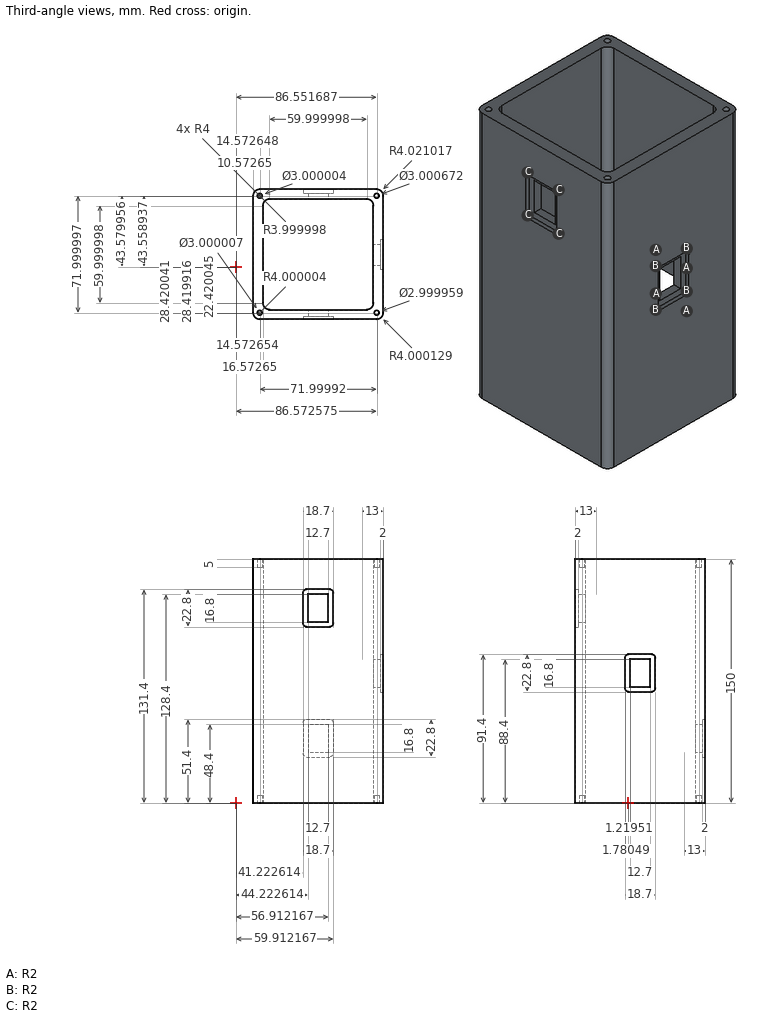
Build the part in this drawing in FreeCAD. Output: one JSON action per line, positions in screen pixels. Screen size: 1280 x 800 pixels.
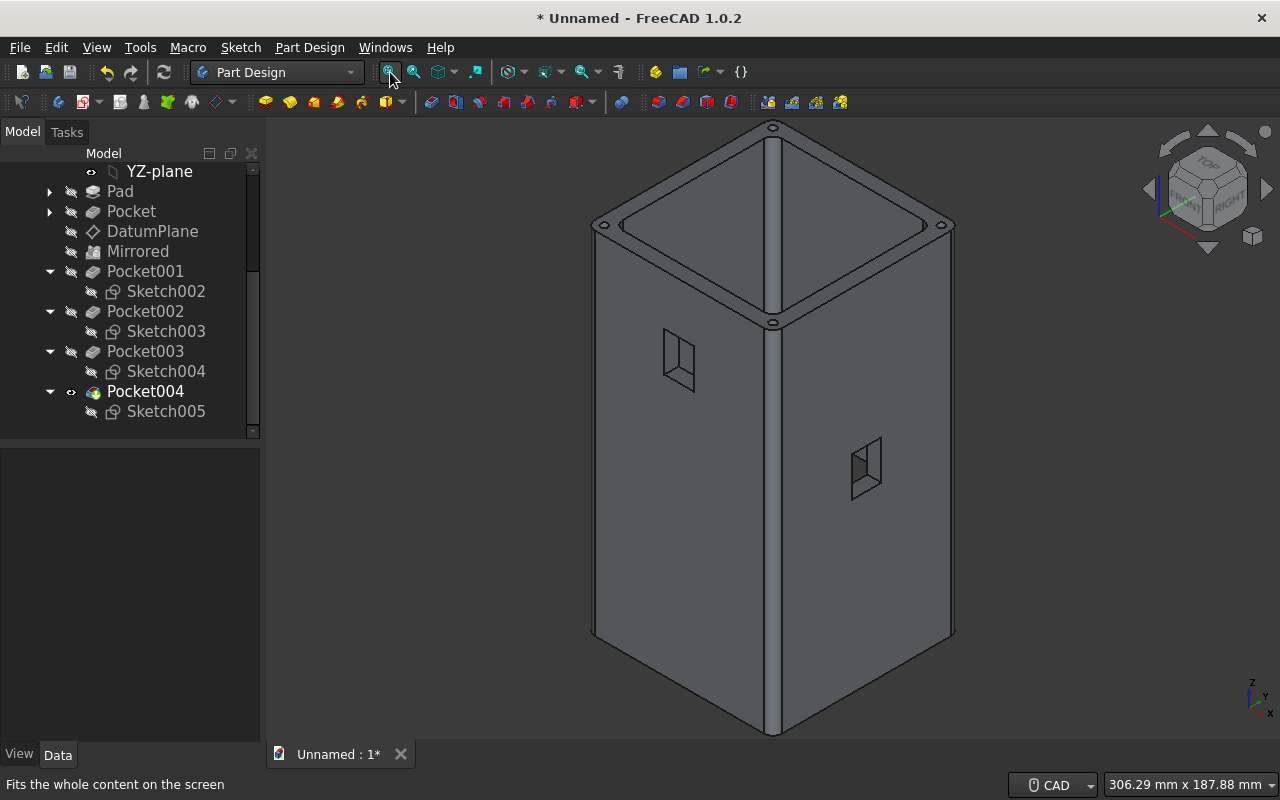
{"action": "key", "text": "v f"}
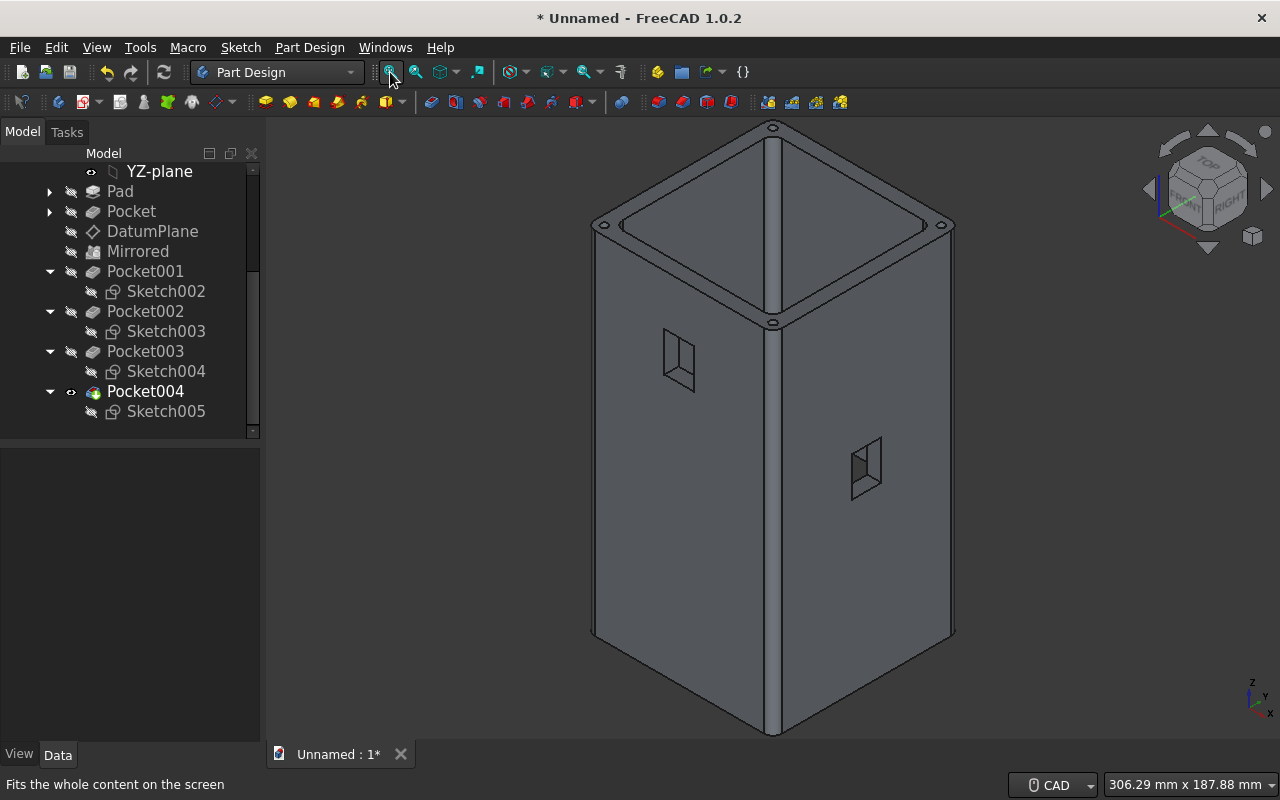
{"action": "scroll", "coordinate": [886, 512], "scroll_direction": "up", "scroll_amount": 9}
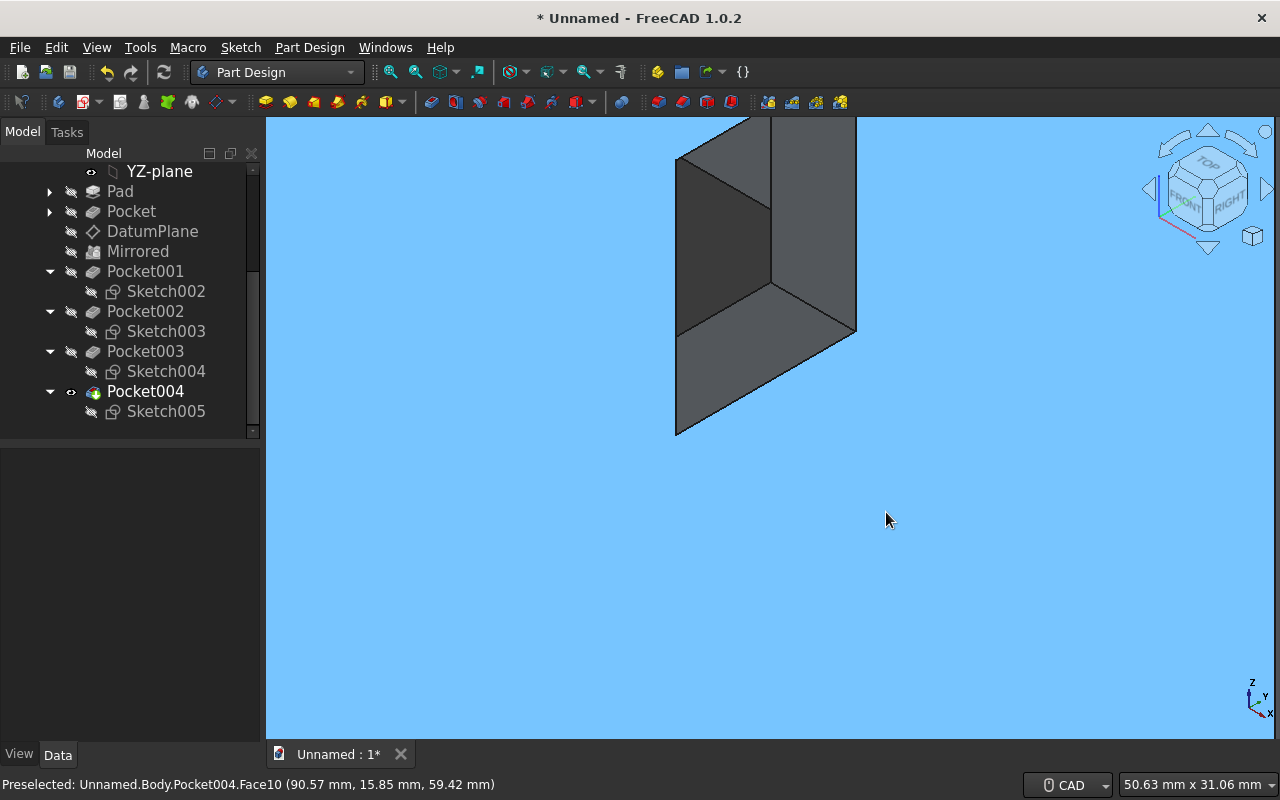
{"action": "left_click", "coordinate": [392, 72]}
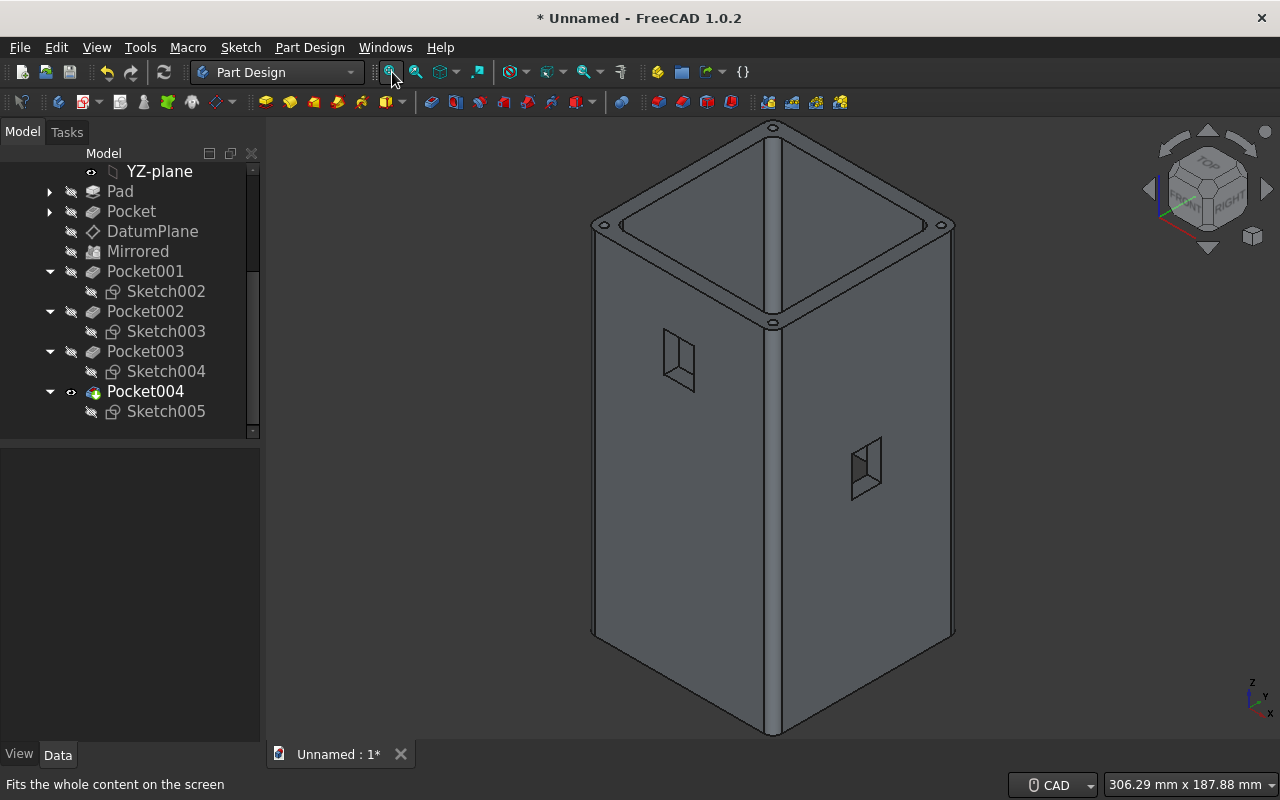
{"action": "key", "text": "2"}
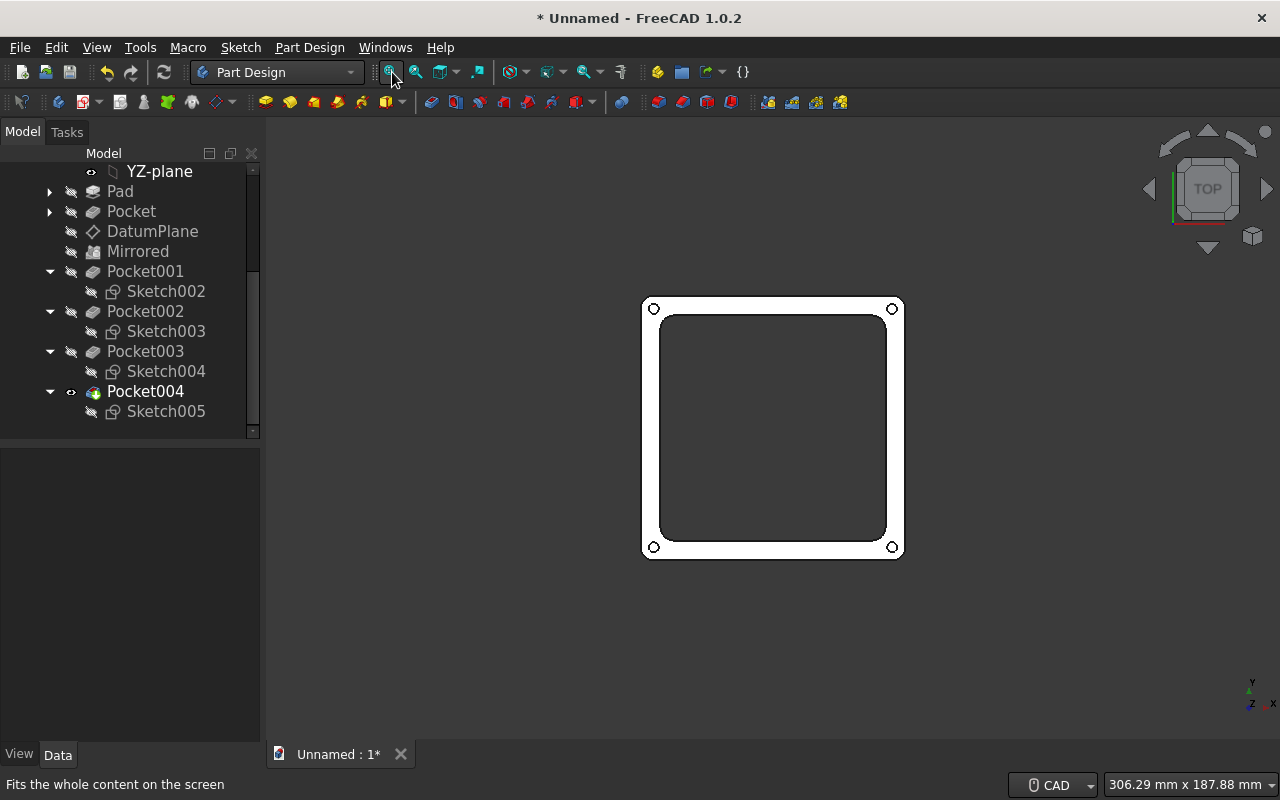
{"action": "left_click", "coordinate": [392, 72]}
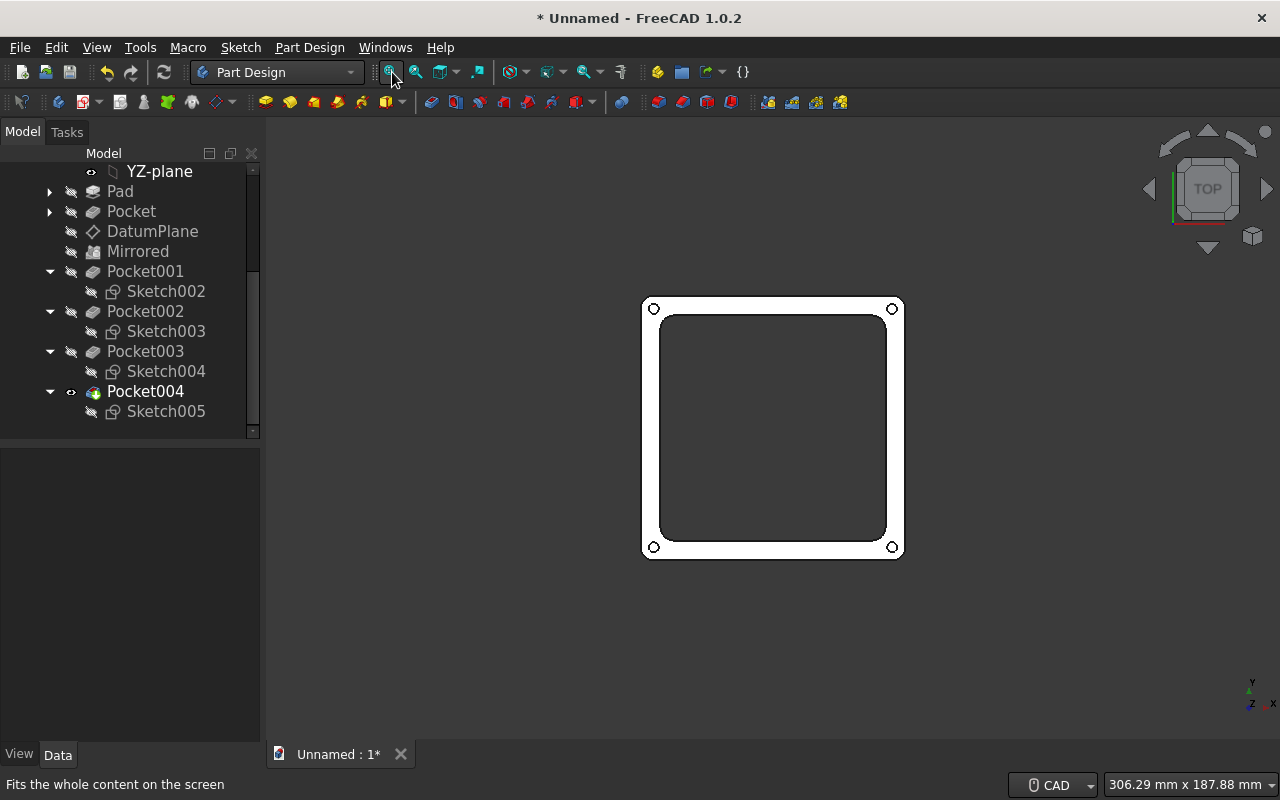
{"action": "scroll", "coordinate": [804, 298], "scroll_direction": "up", "scroll_amount": 9}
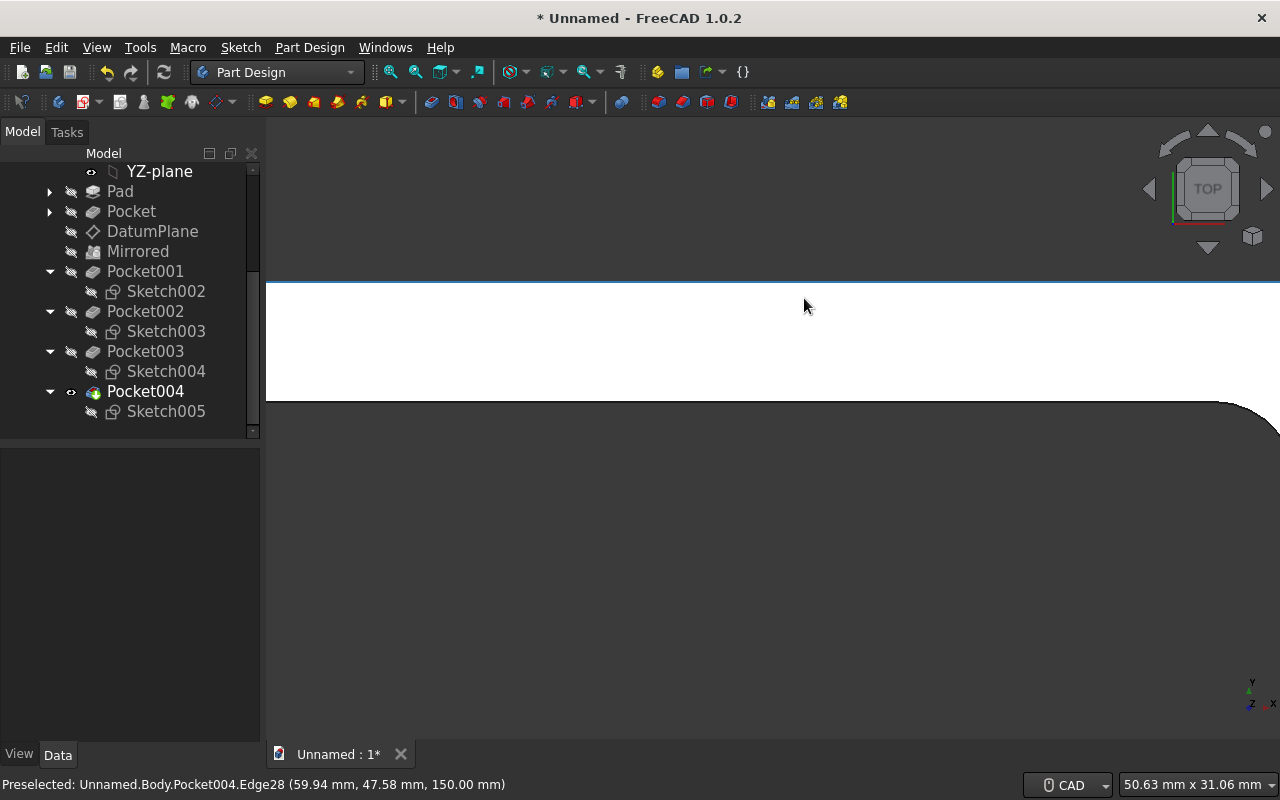
{"action": "left_click", "coordinate": [392, 72]}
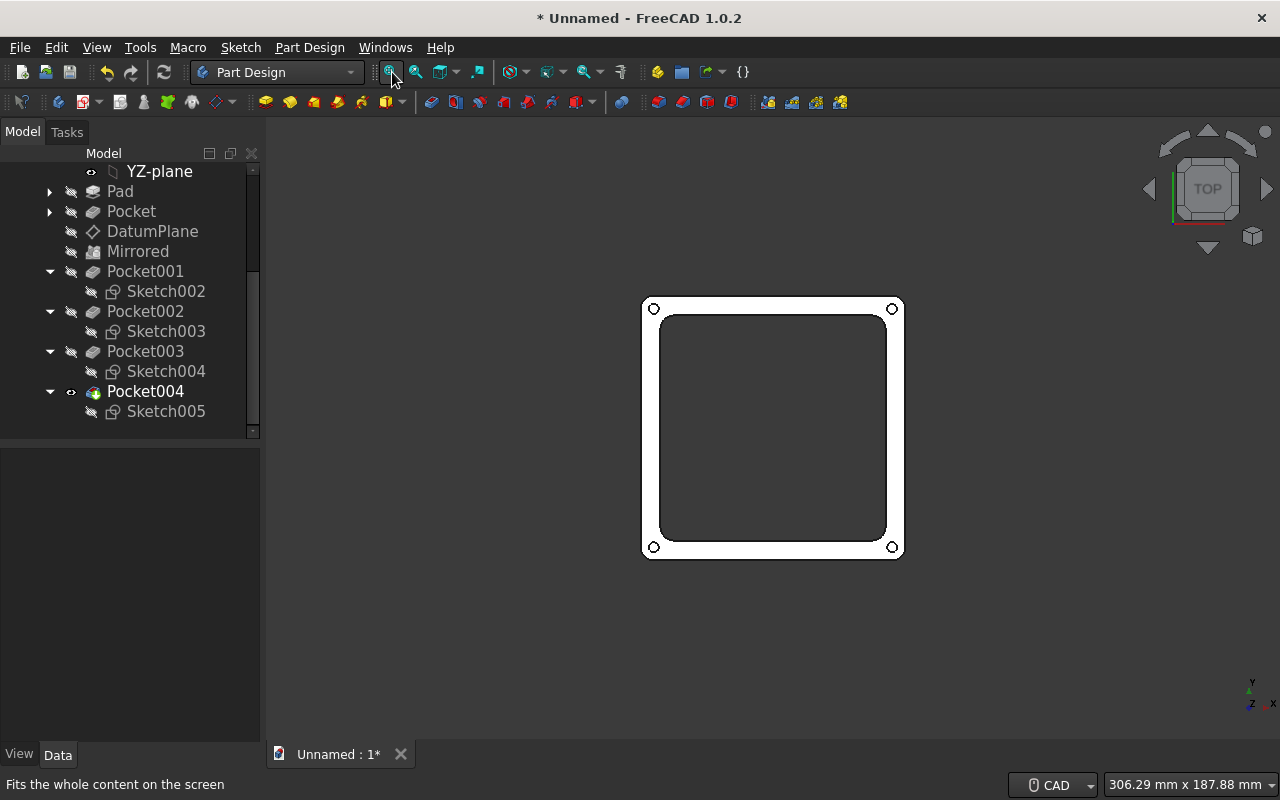
{"action": "key", "text": "1"}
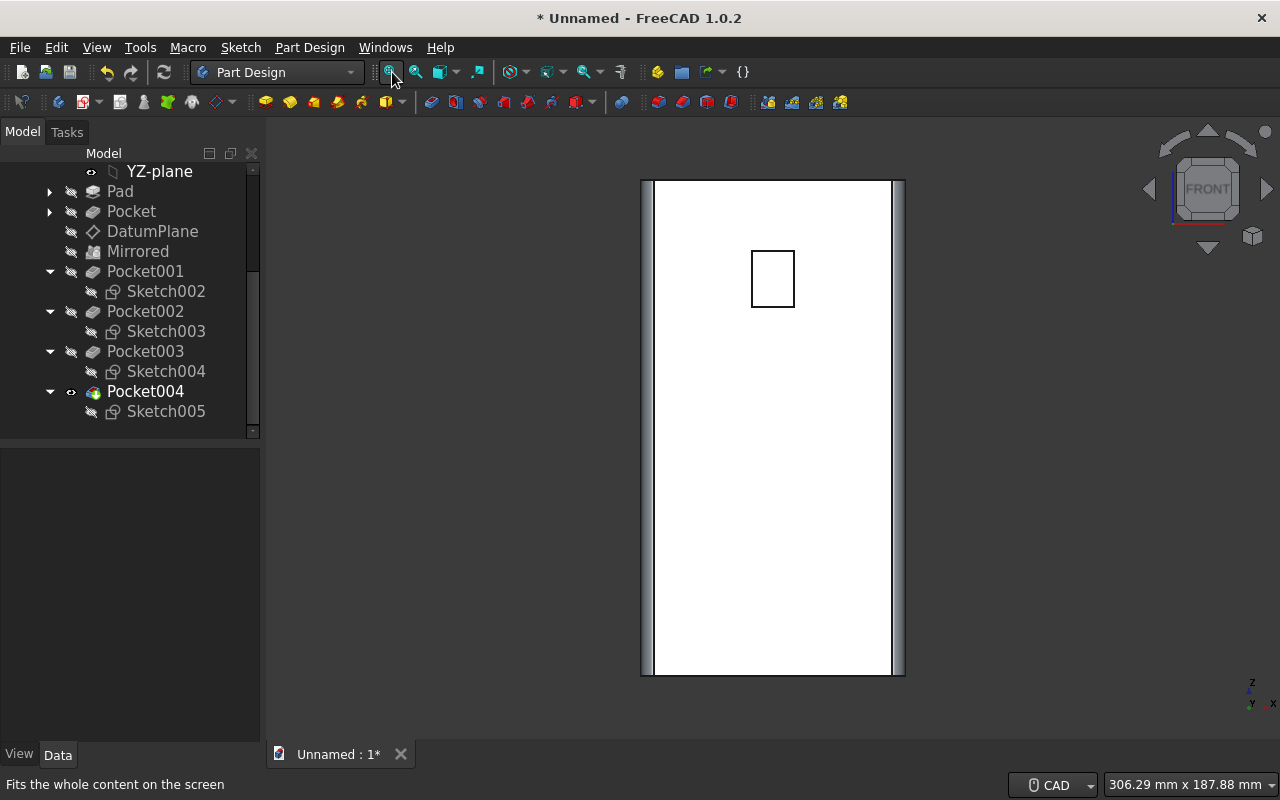
{"action": "scroll", "coordinate": [804, 581], "scroll_direction": "up", "scroll_amount": 9}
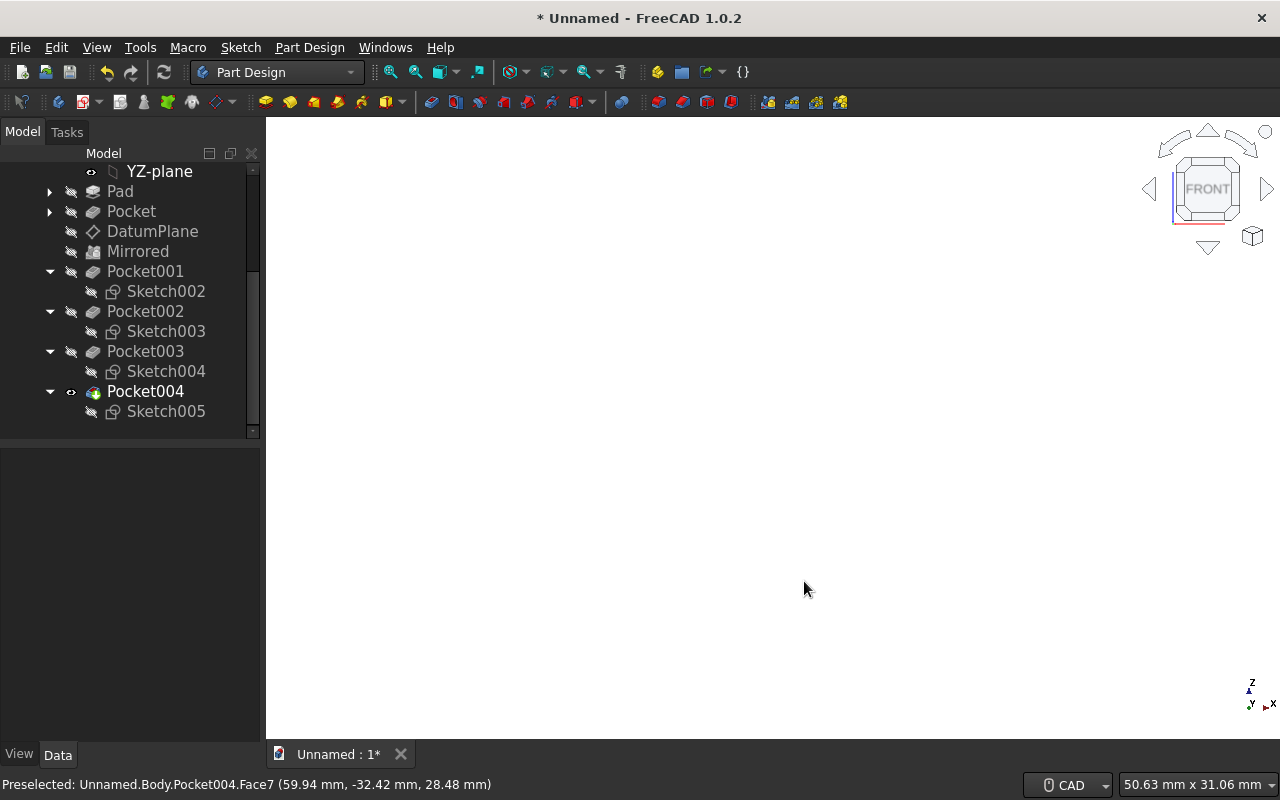
{"action": "key", "text": "v f"}